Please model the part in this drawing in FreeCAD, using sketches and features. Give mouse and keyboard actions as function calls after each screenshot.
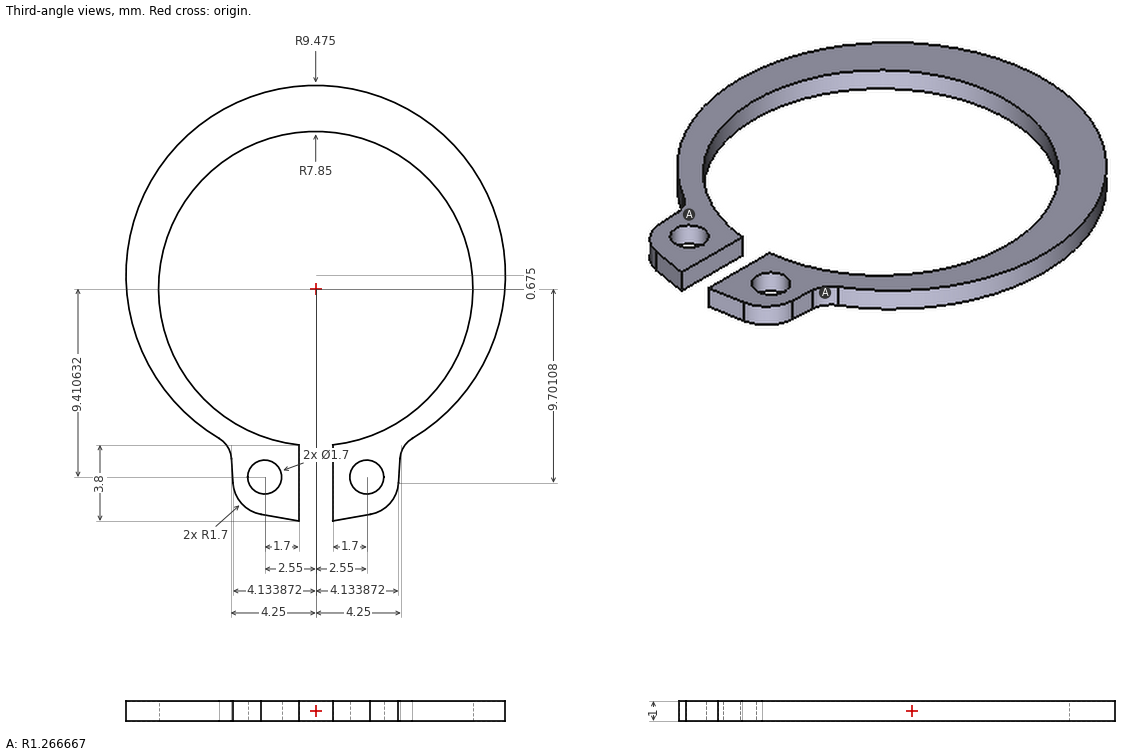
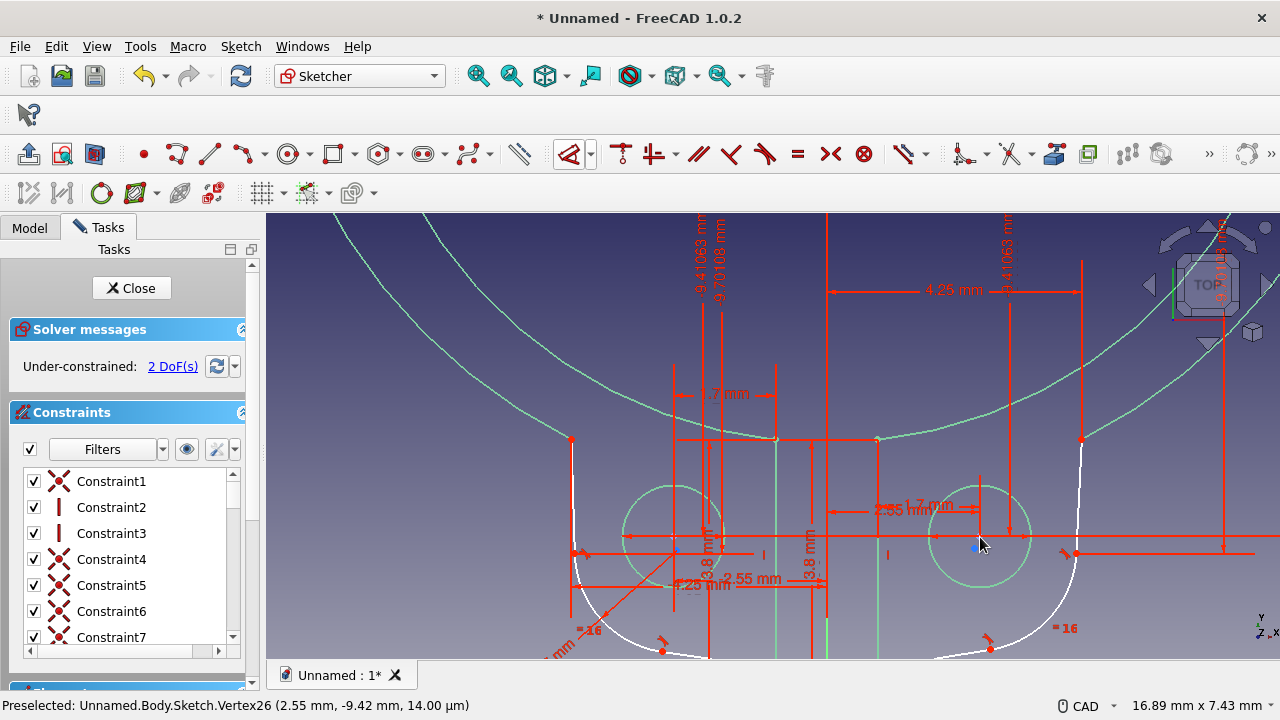
scroll(674, 542, down, 8)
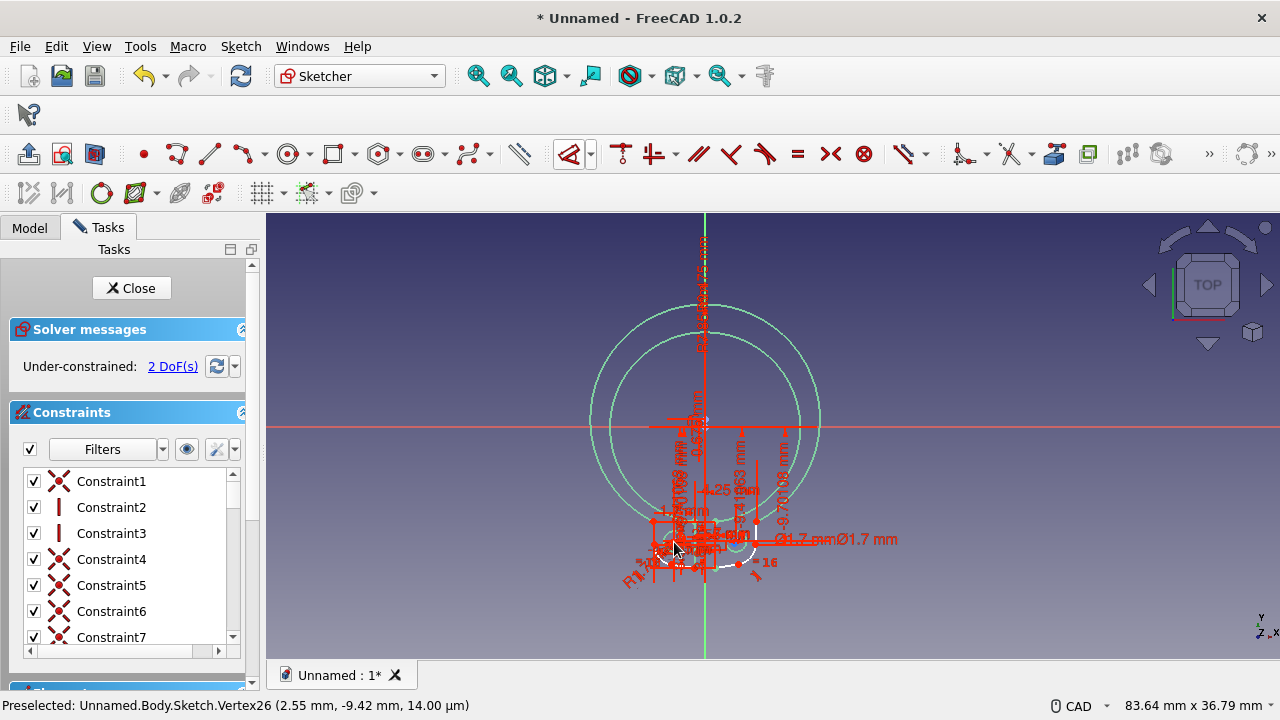
click(756, 545)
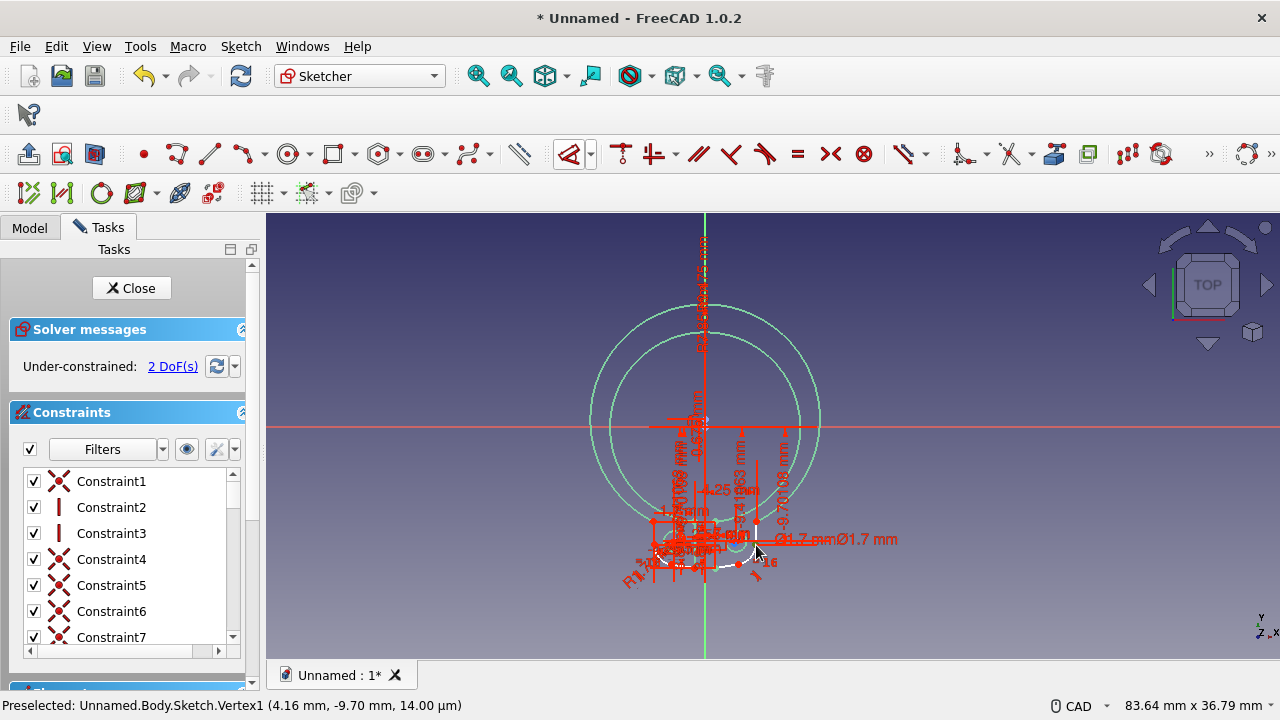
click(590, 154)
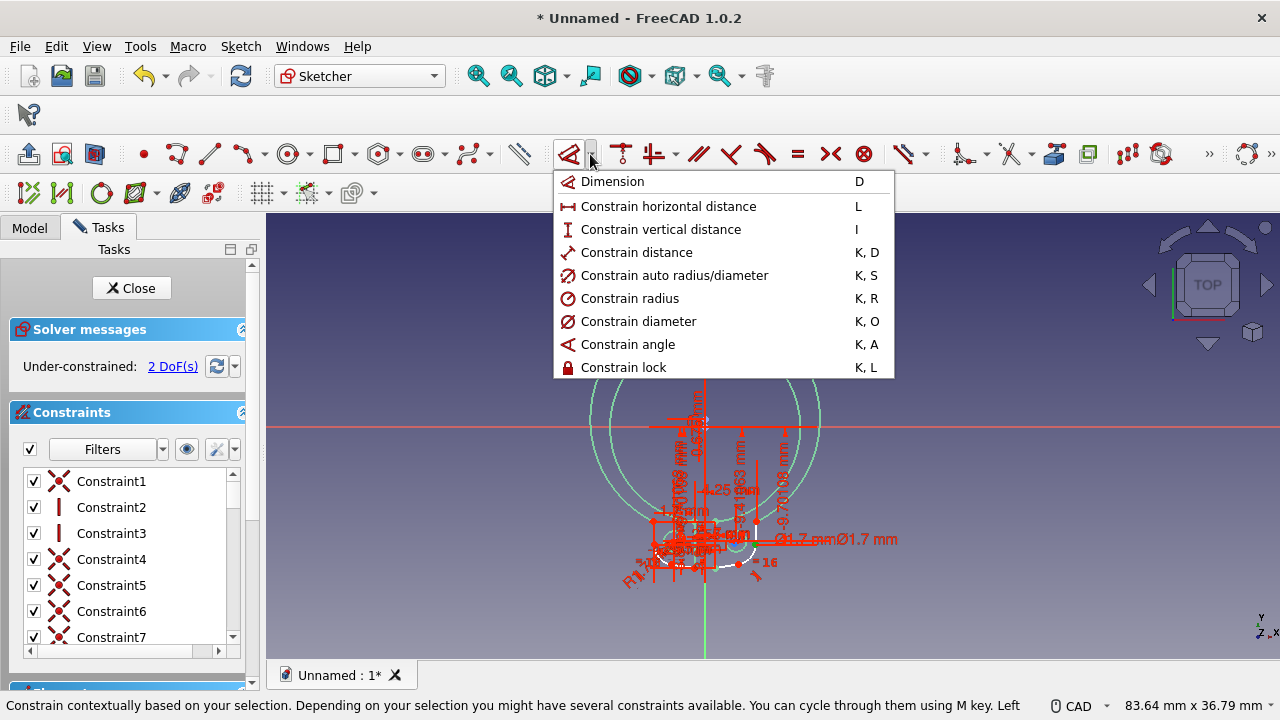
click(724, 206)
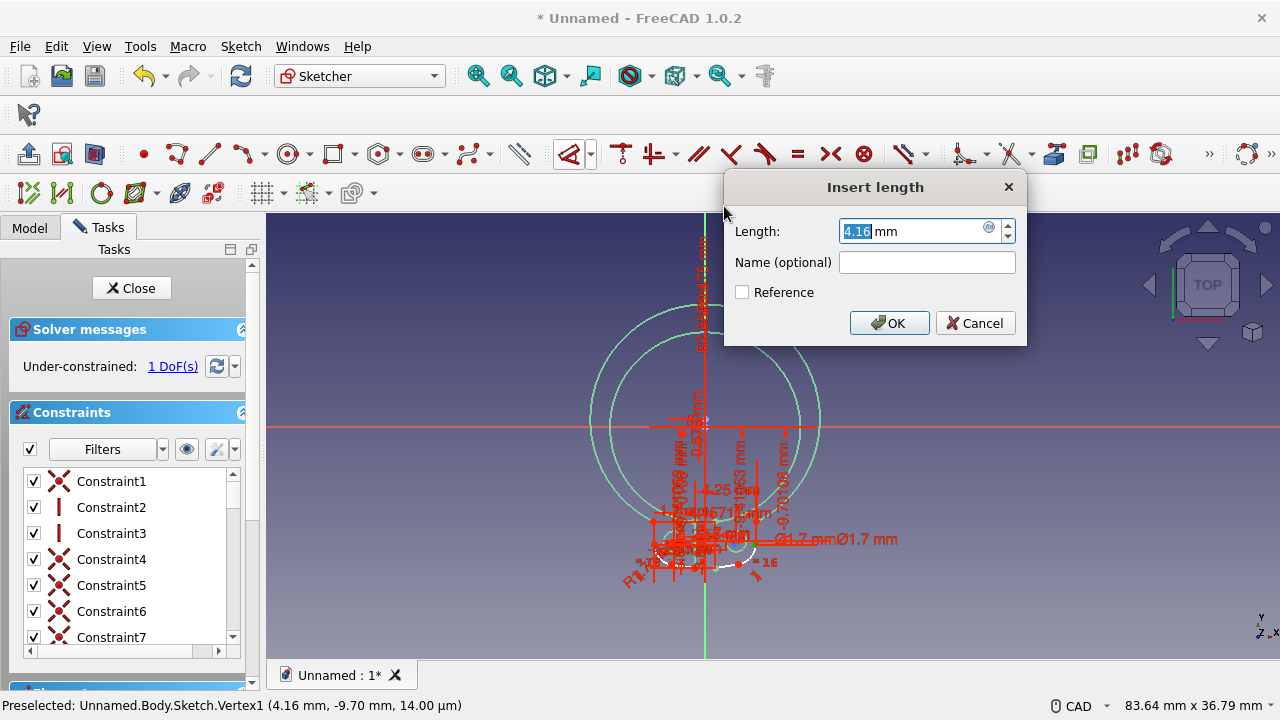
text(4.133872)
key(Return)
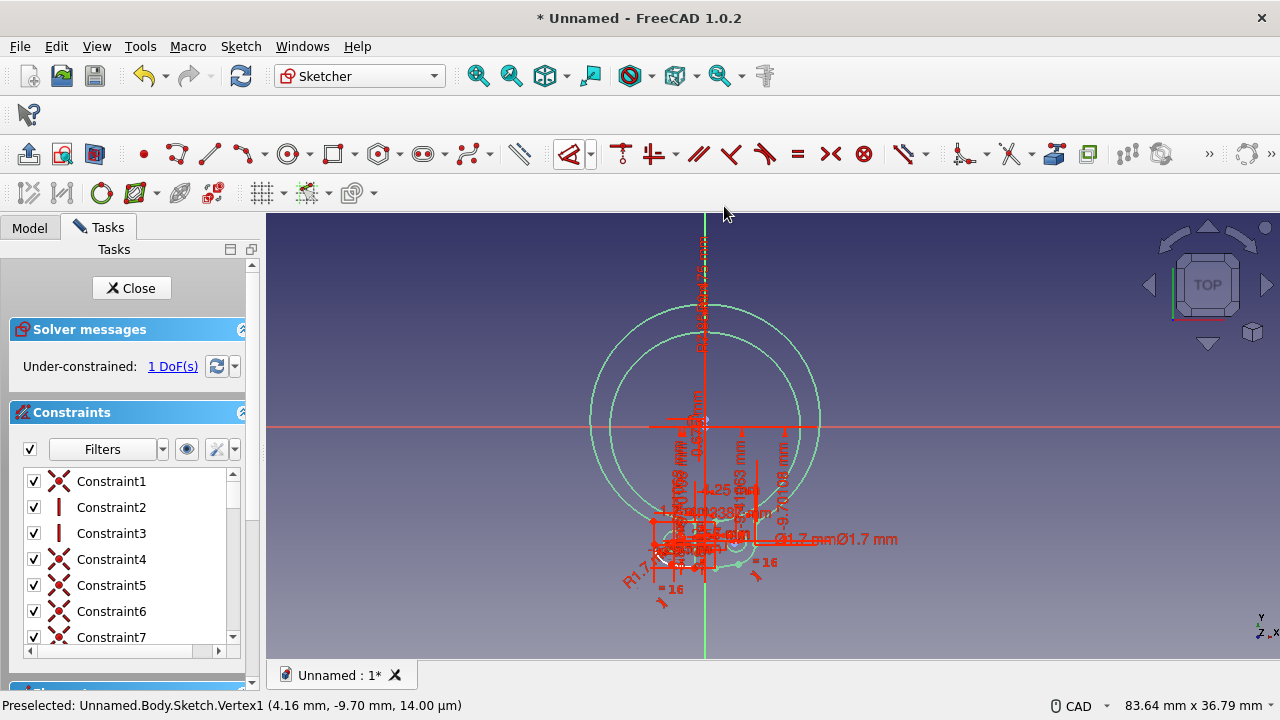
click(654, 545)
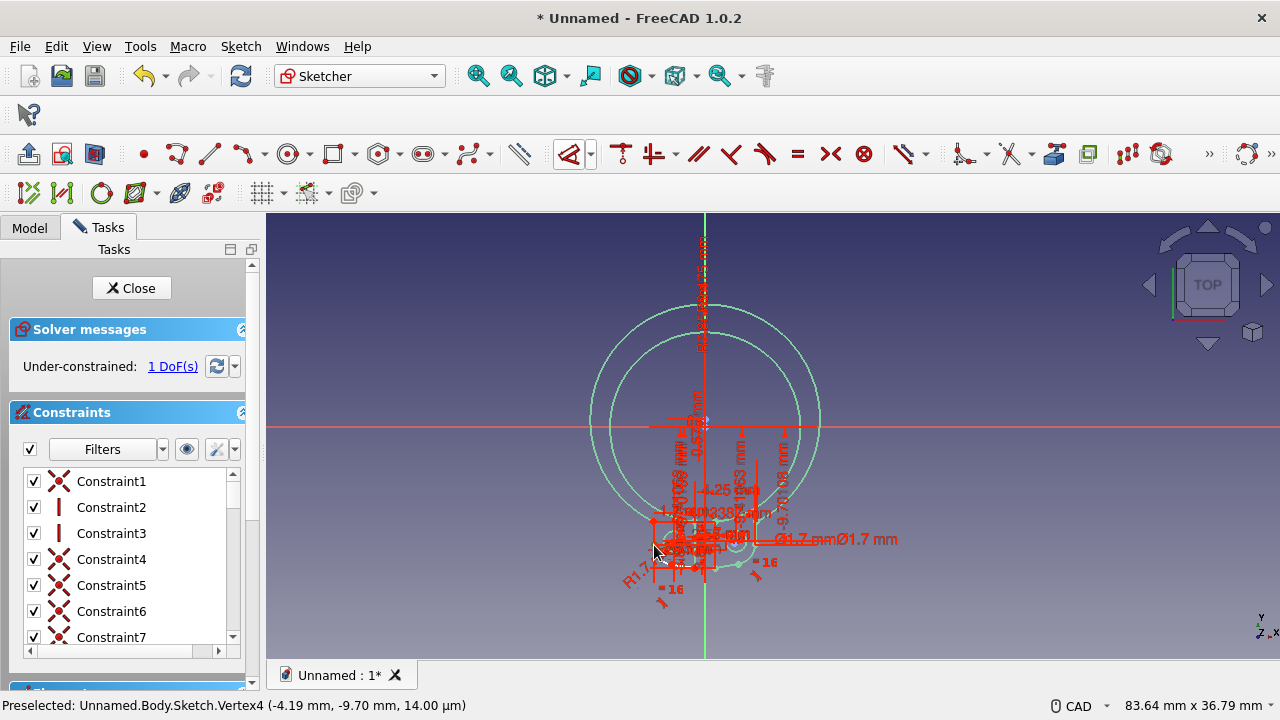
key(l)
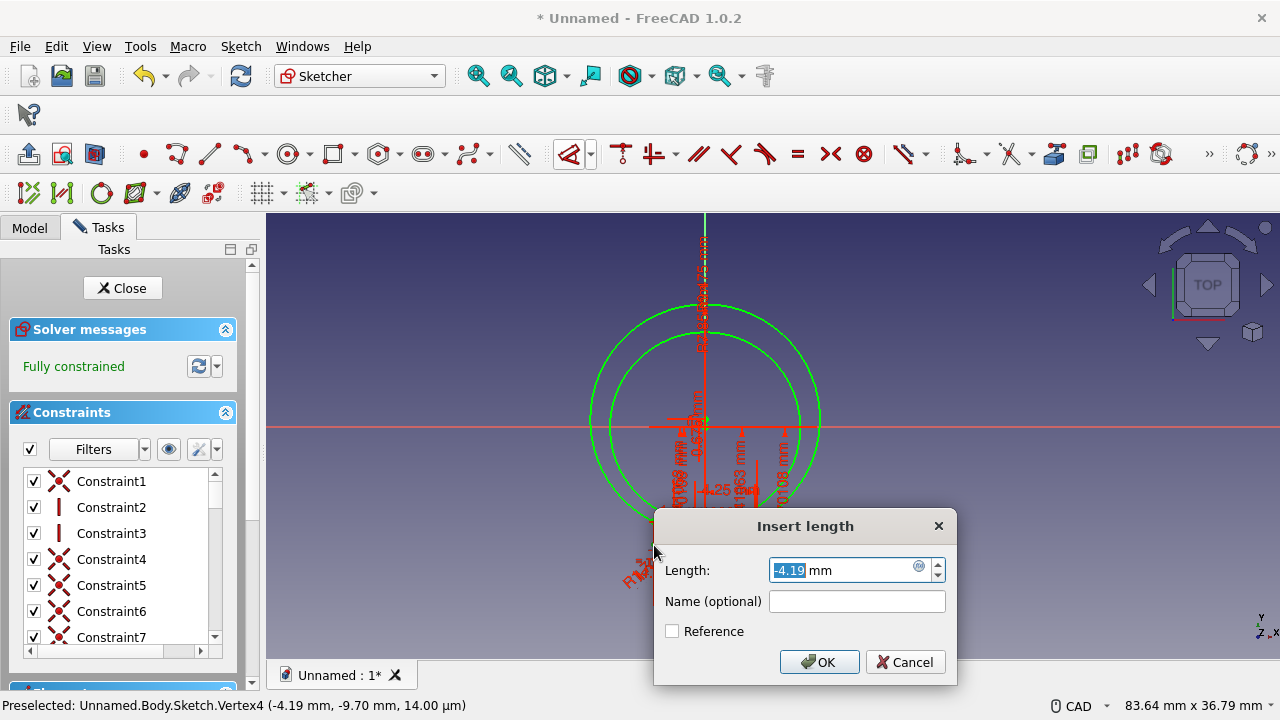
text(-4.133872)
key(Return)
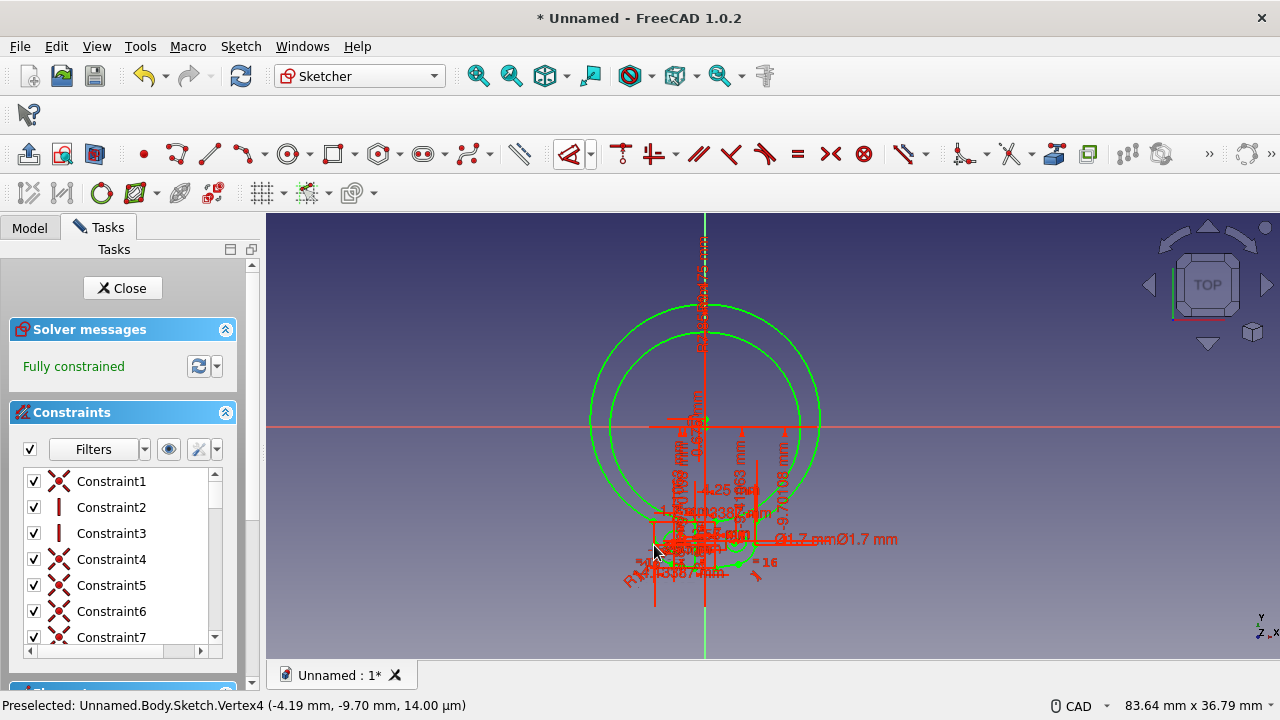
click(123, 288)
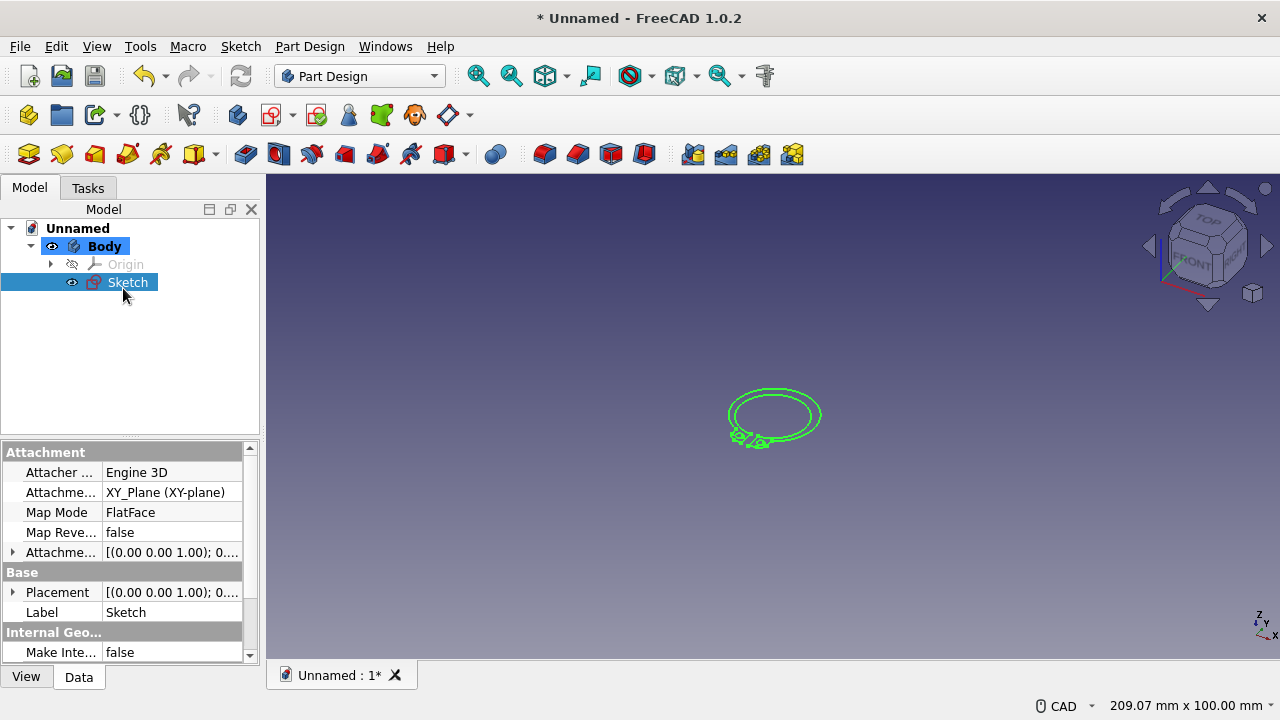
click(29, 154)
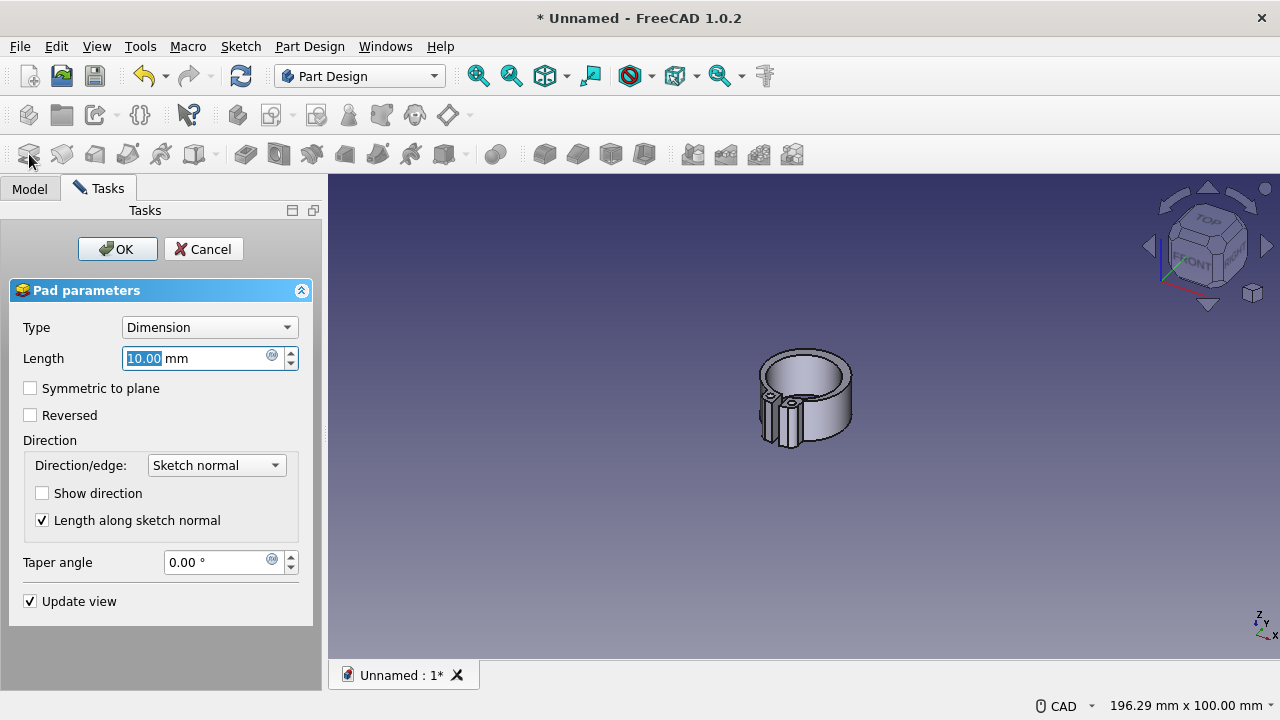
text(1)
key(Tab)